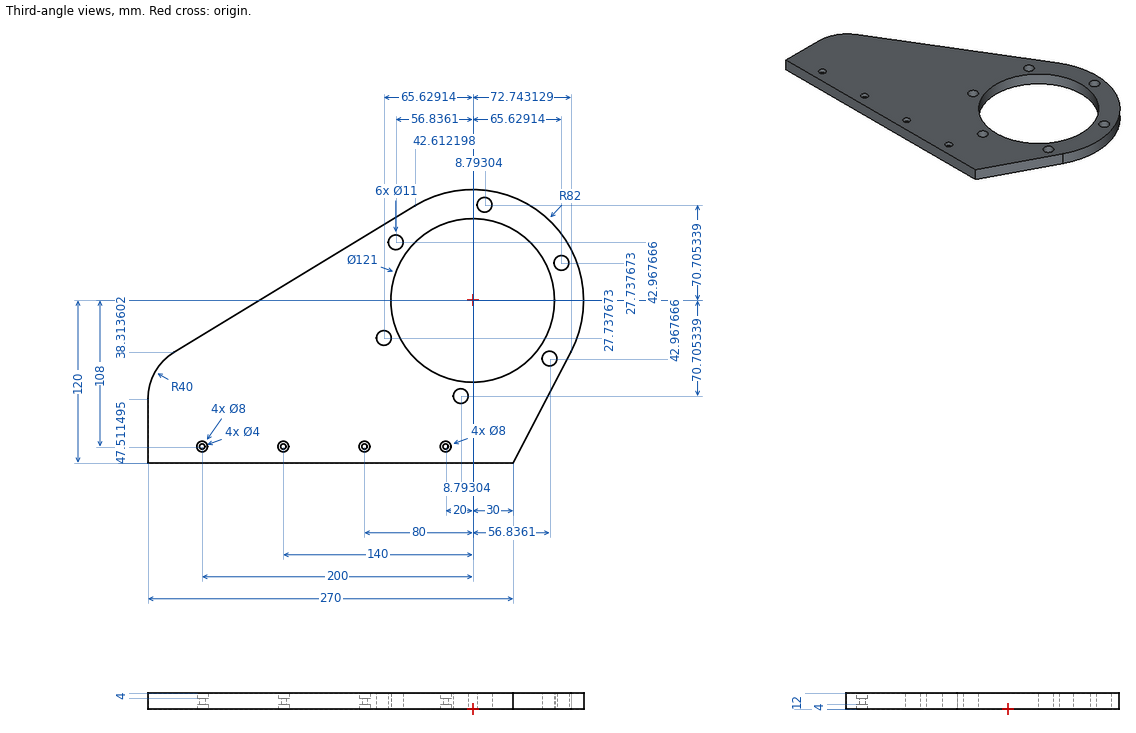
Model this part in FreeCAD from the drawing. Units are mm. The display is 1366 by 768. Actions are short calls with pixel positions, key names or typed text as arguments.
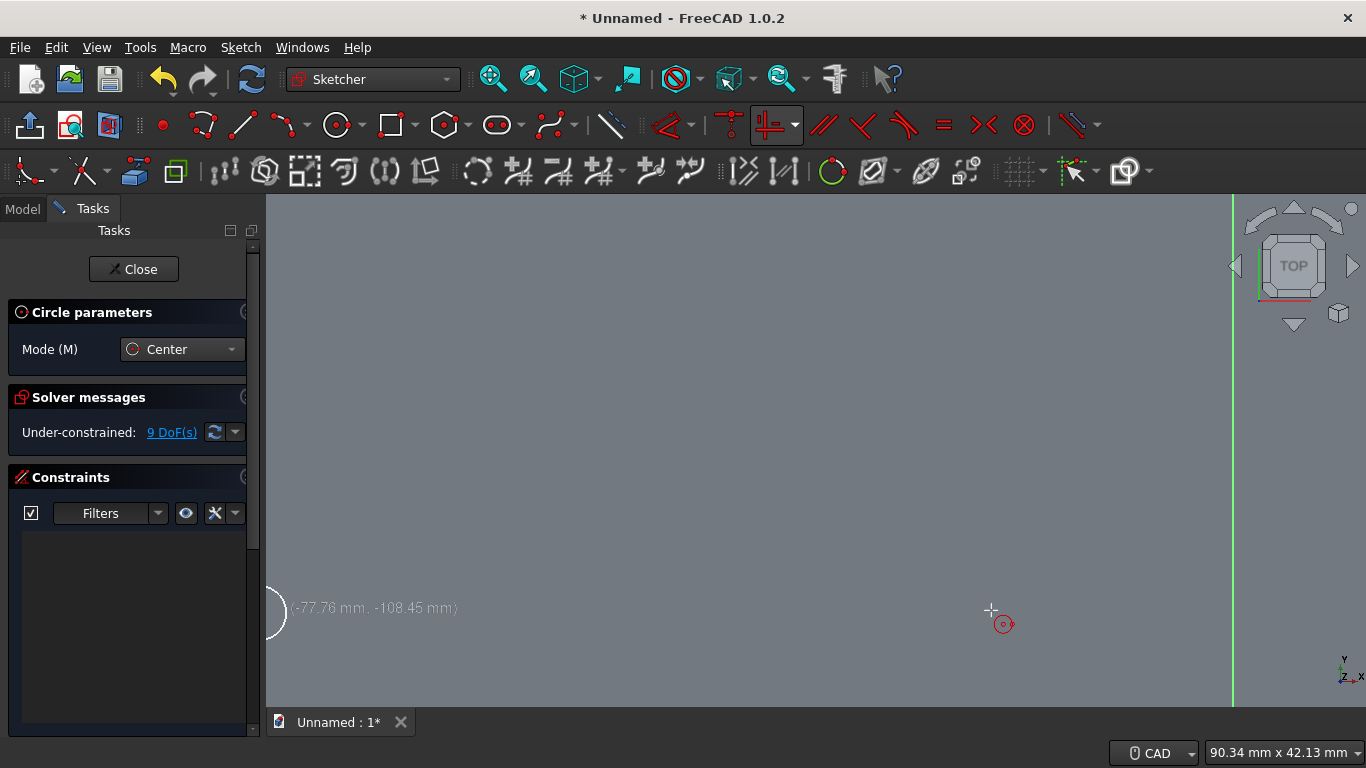
scroll(991, 610, down, 7)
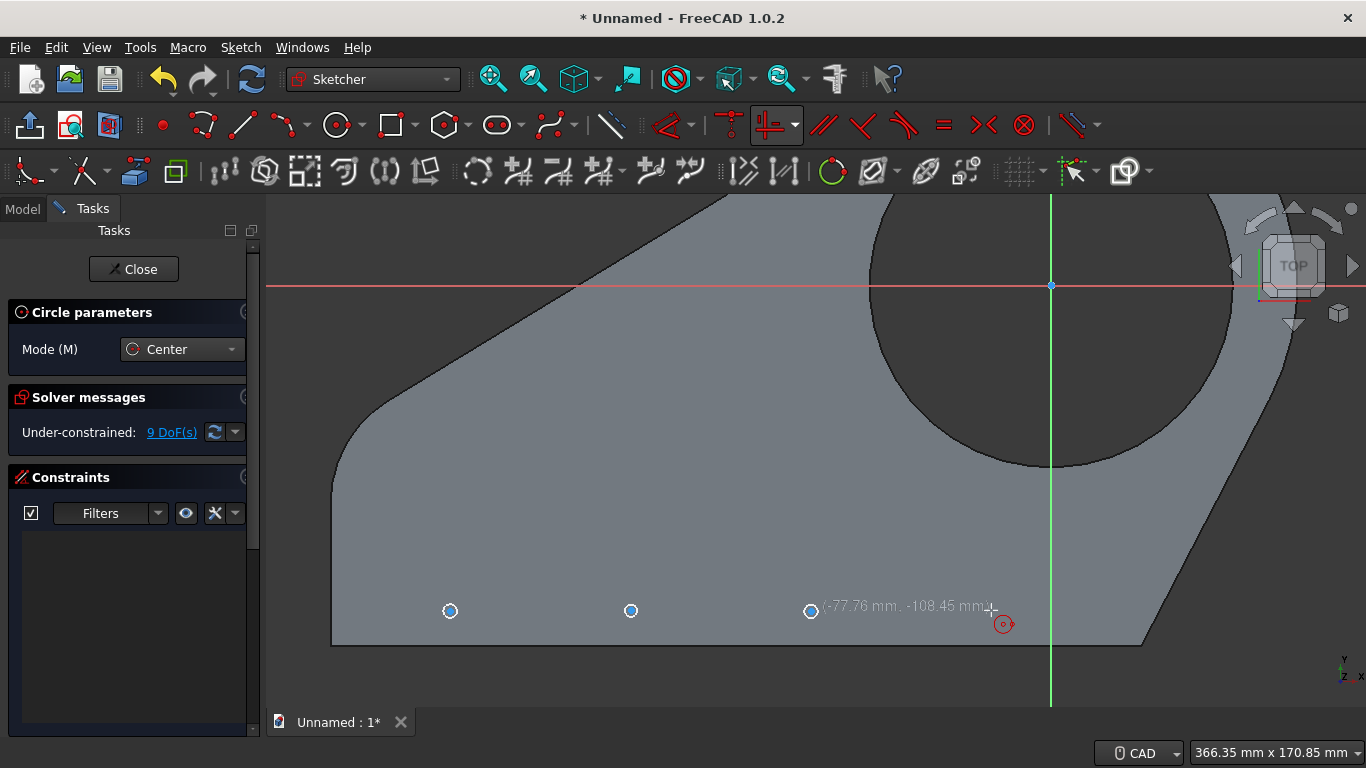
click(991, 610)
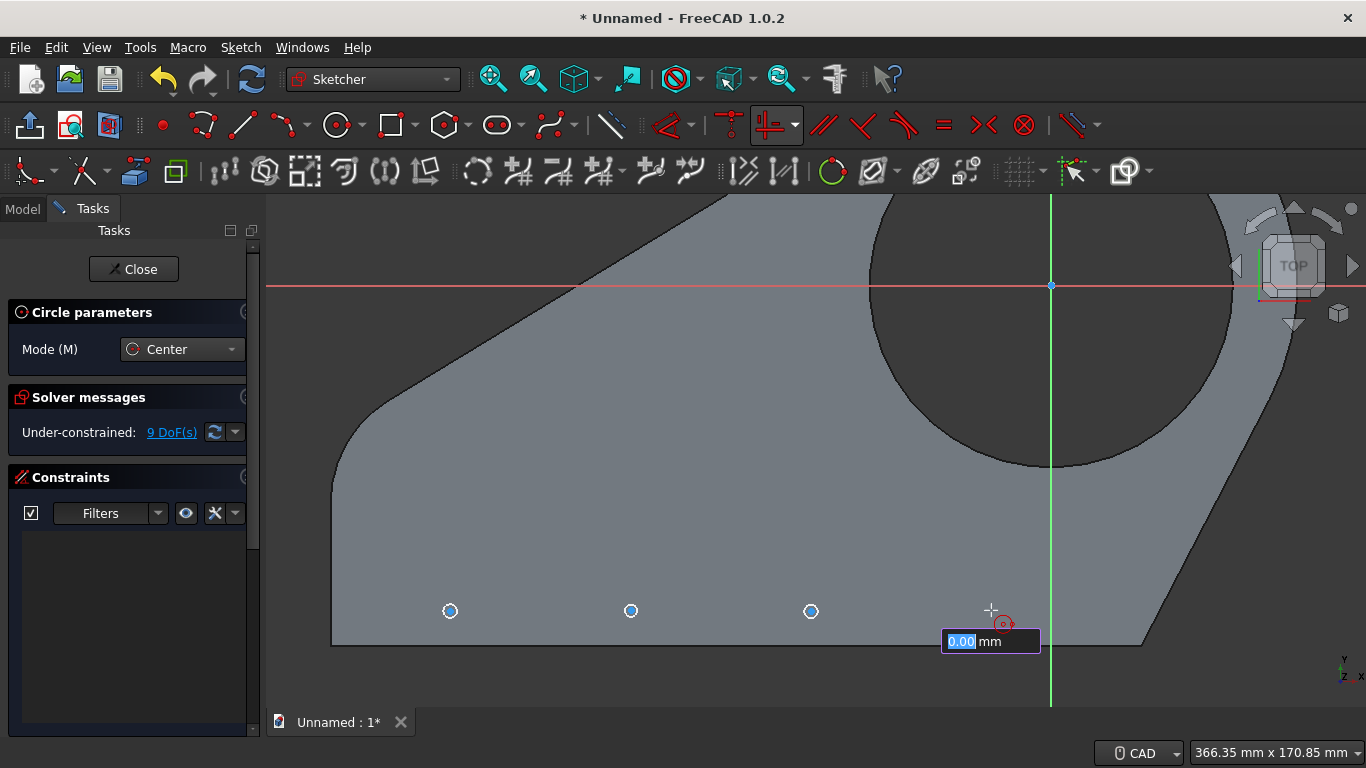
scroll(995, 606, up, 5)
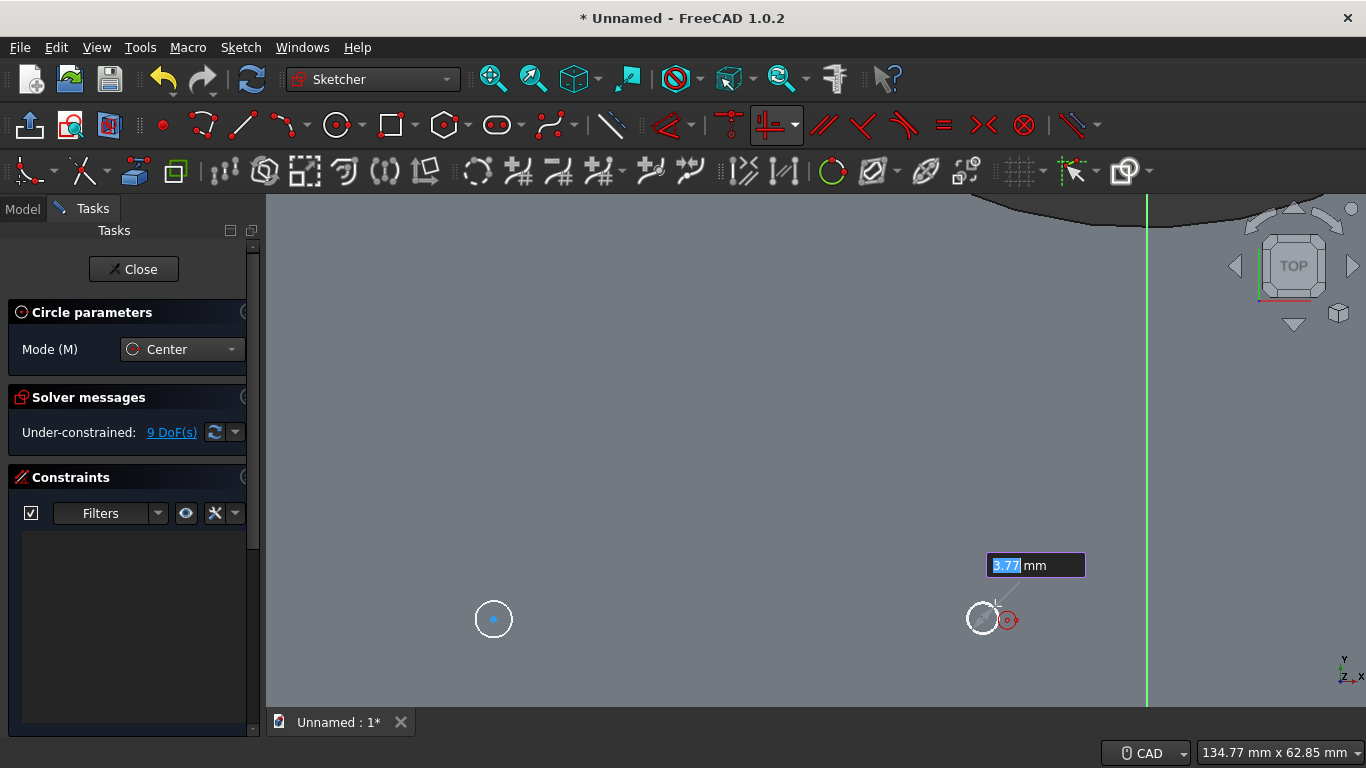
click(995, 604)
key(Escape)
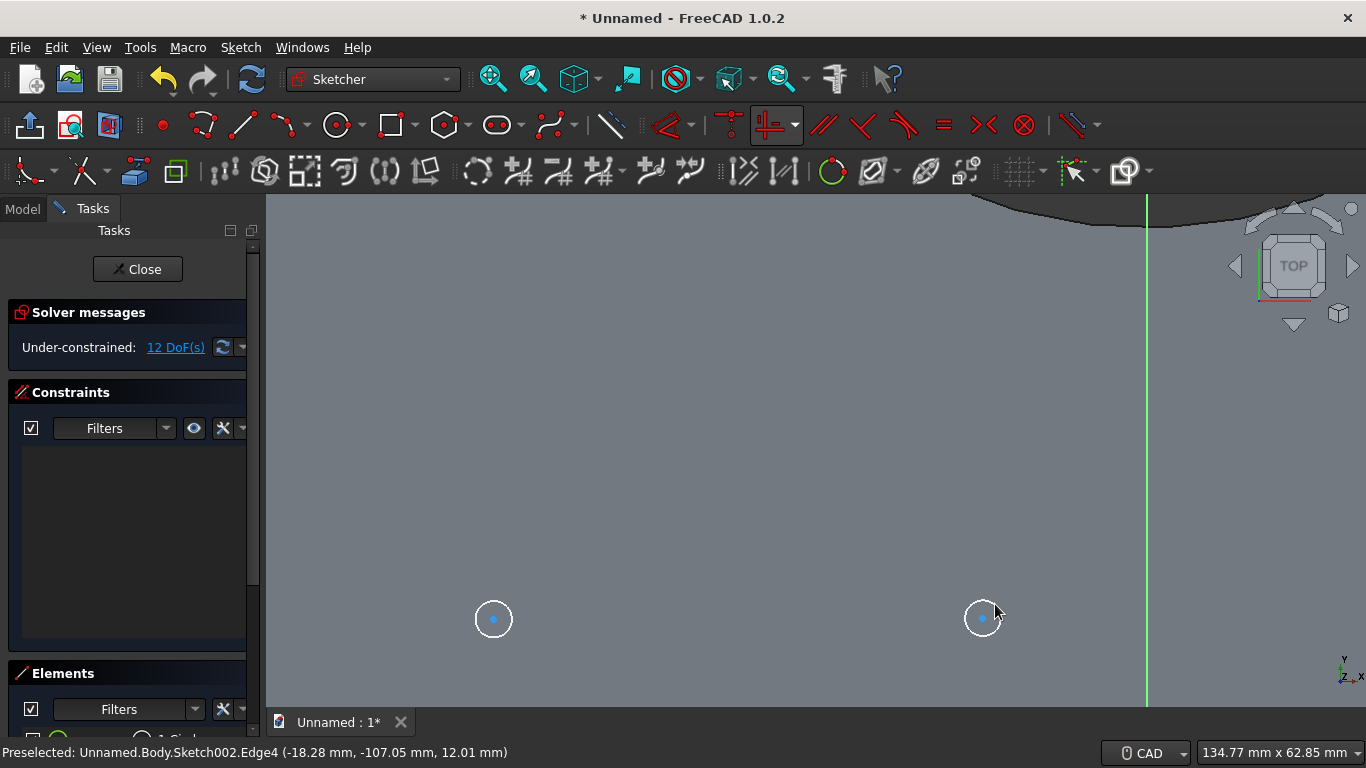
scroll(995, 606, down, 5)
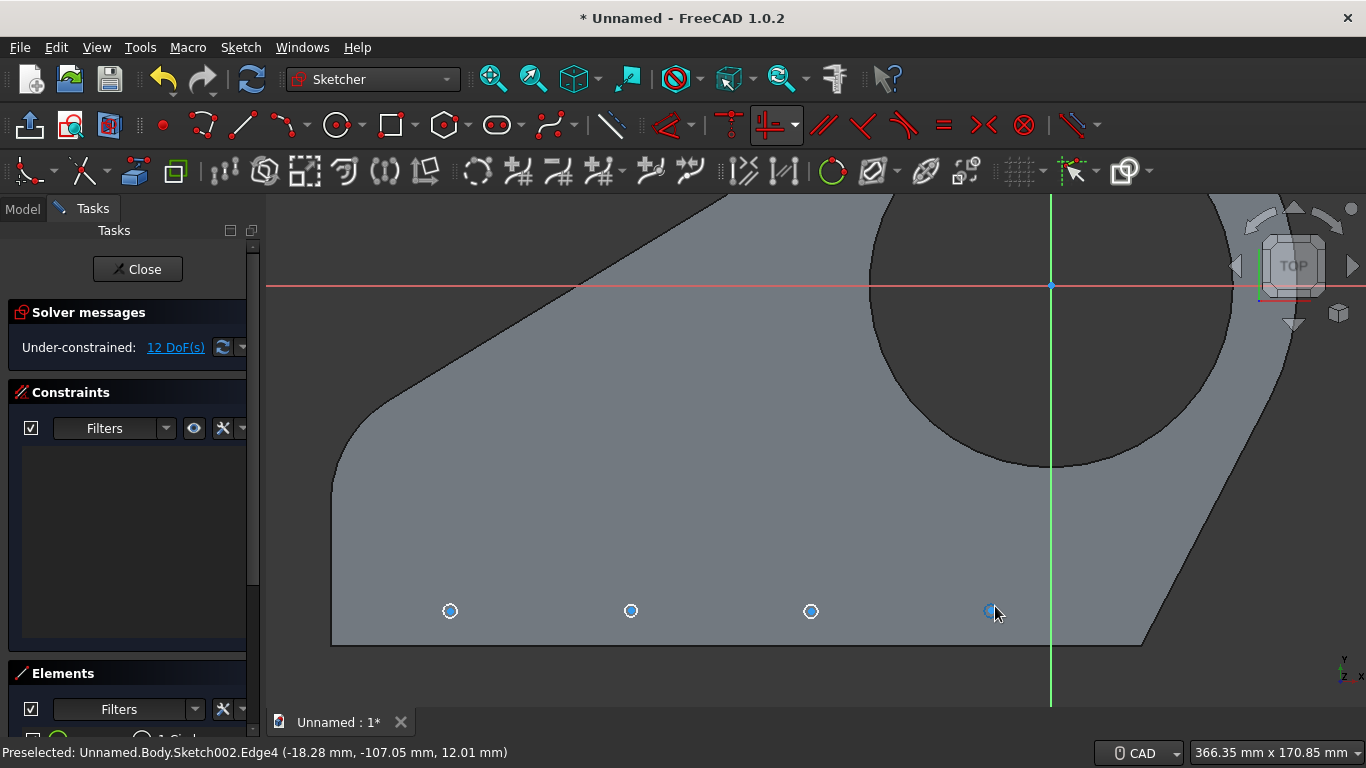
scroll(455, 606, up, 4)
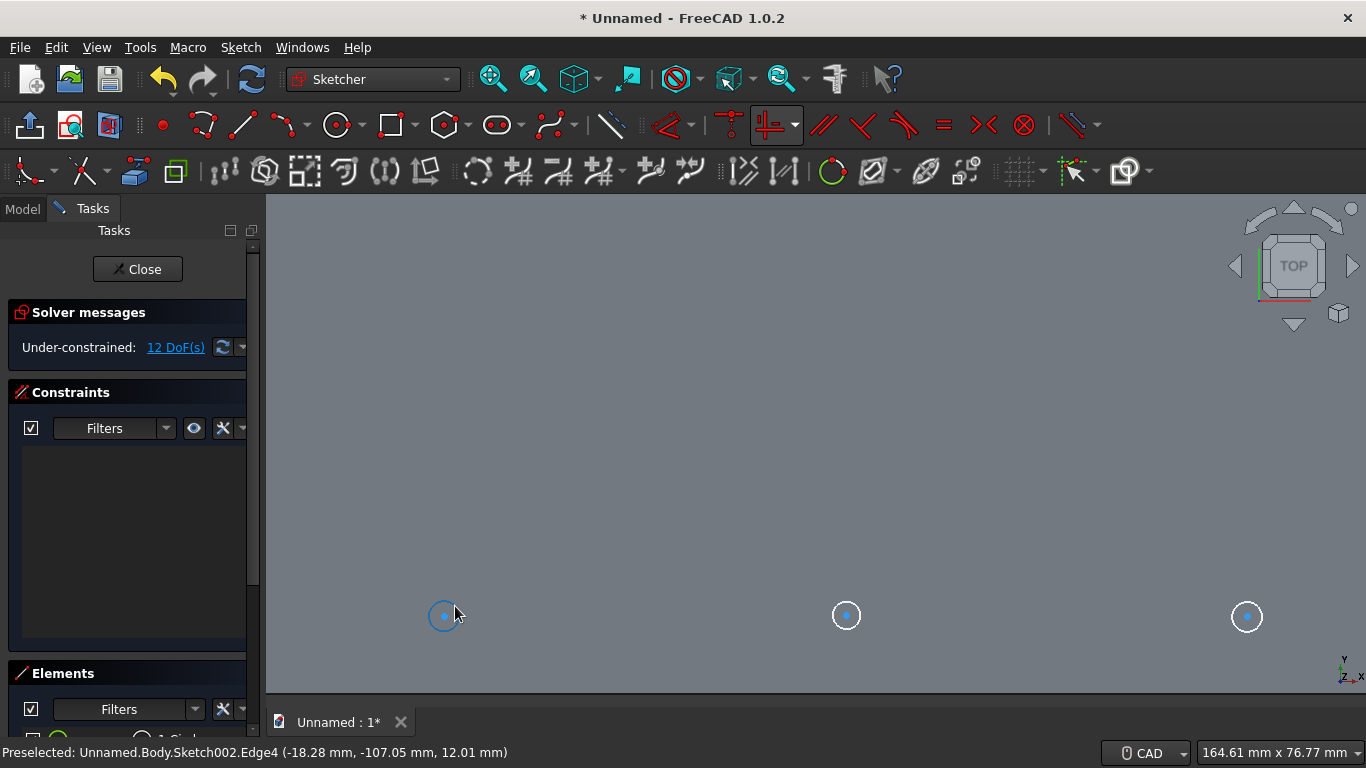
click(455, 606)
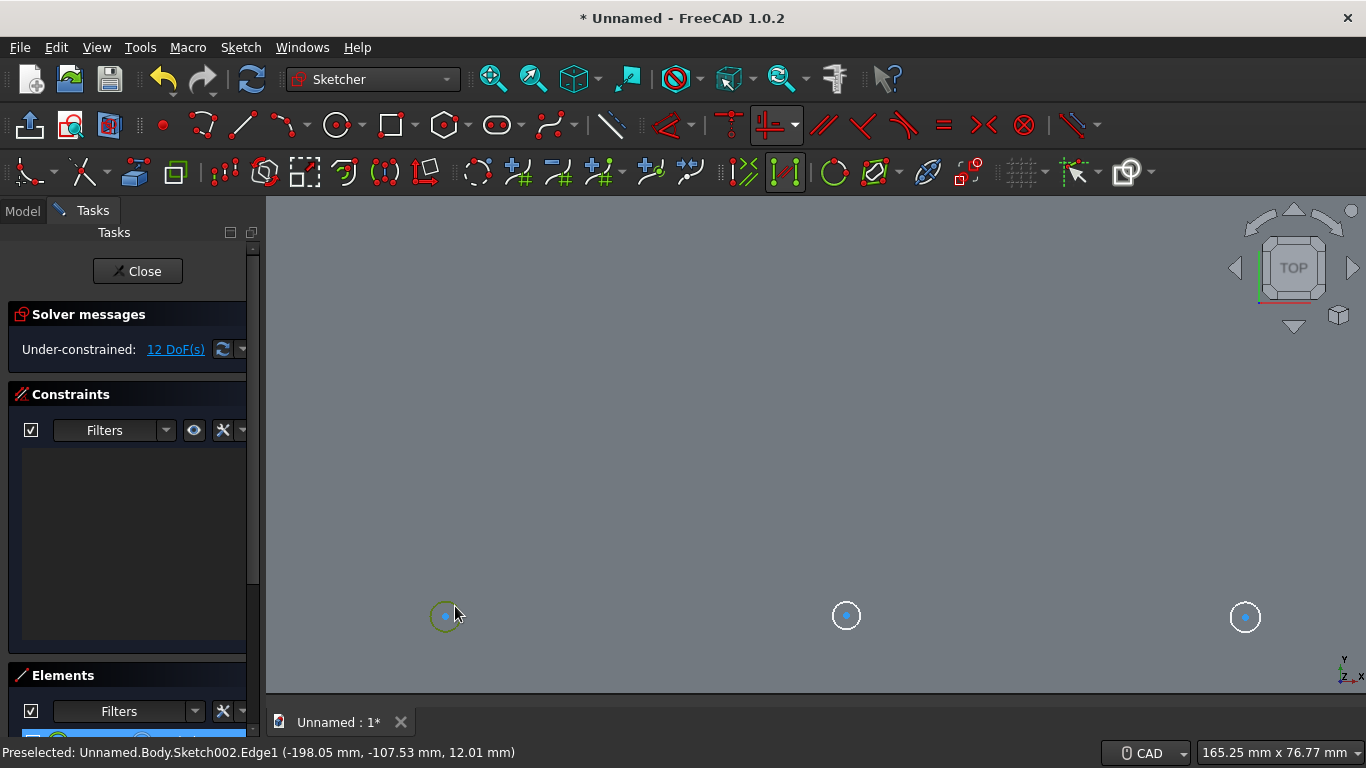
click(856, 606)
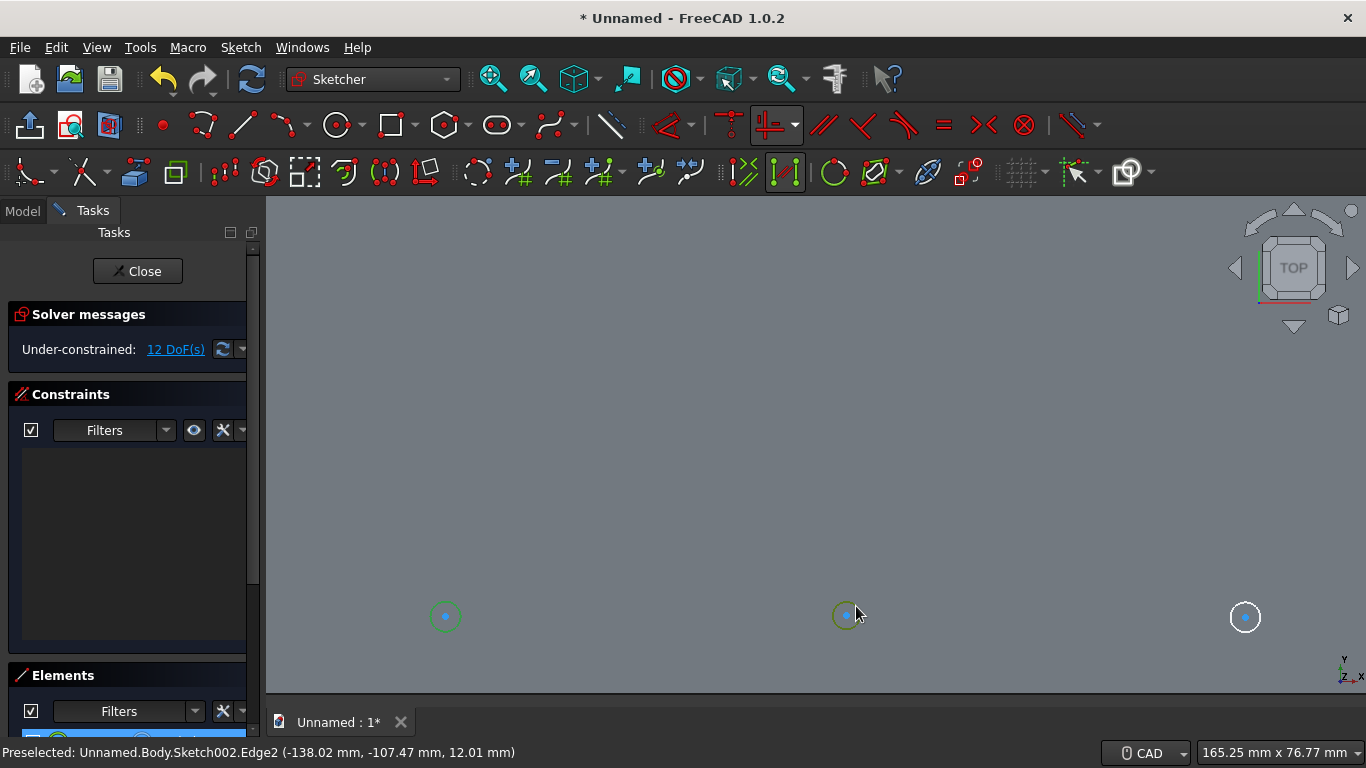
scroll(455, 607, down, 4)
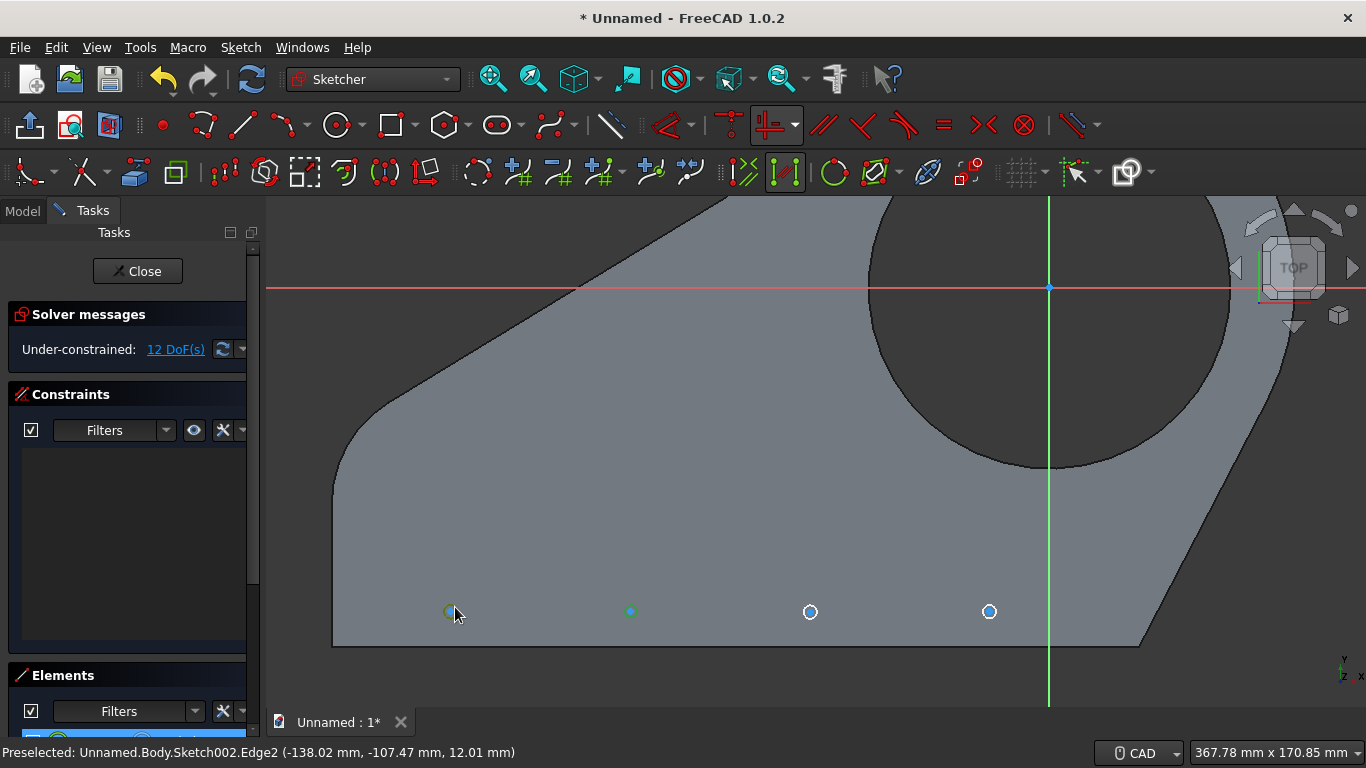
scroll(815, 607, up, 4)